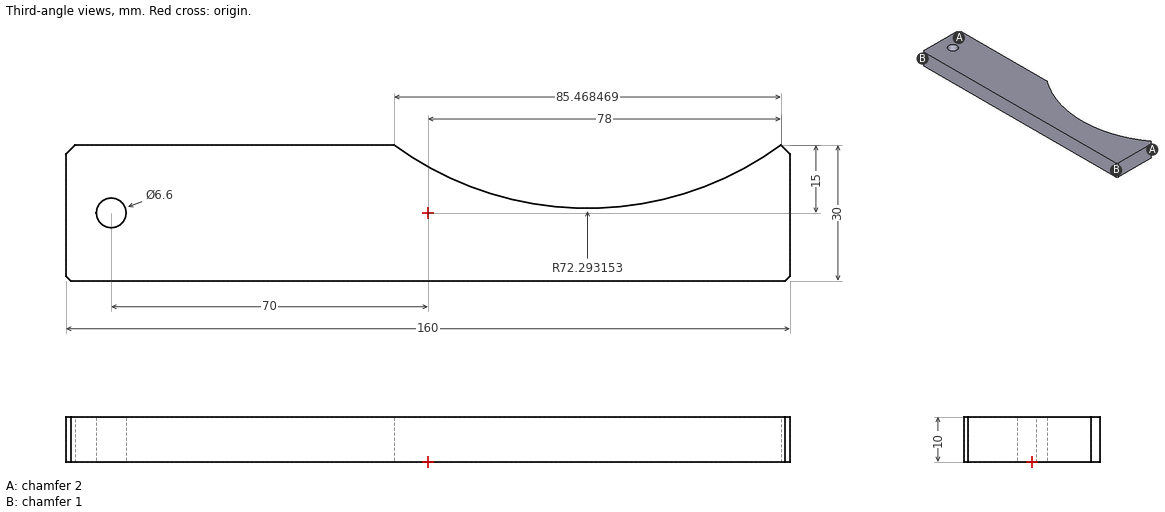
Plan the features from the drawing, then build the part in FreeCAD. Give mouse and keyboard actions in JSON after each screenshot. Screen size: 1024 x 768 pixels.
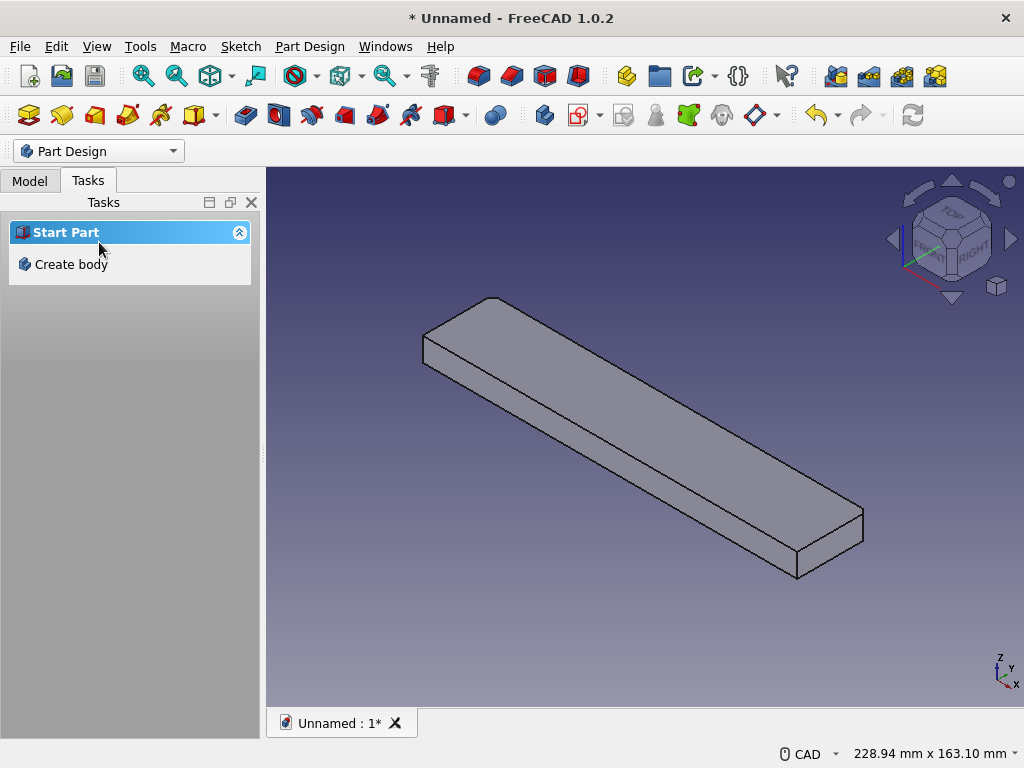
{"action": "left_click", "coordinate": [797, 564]}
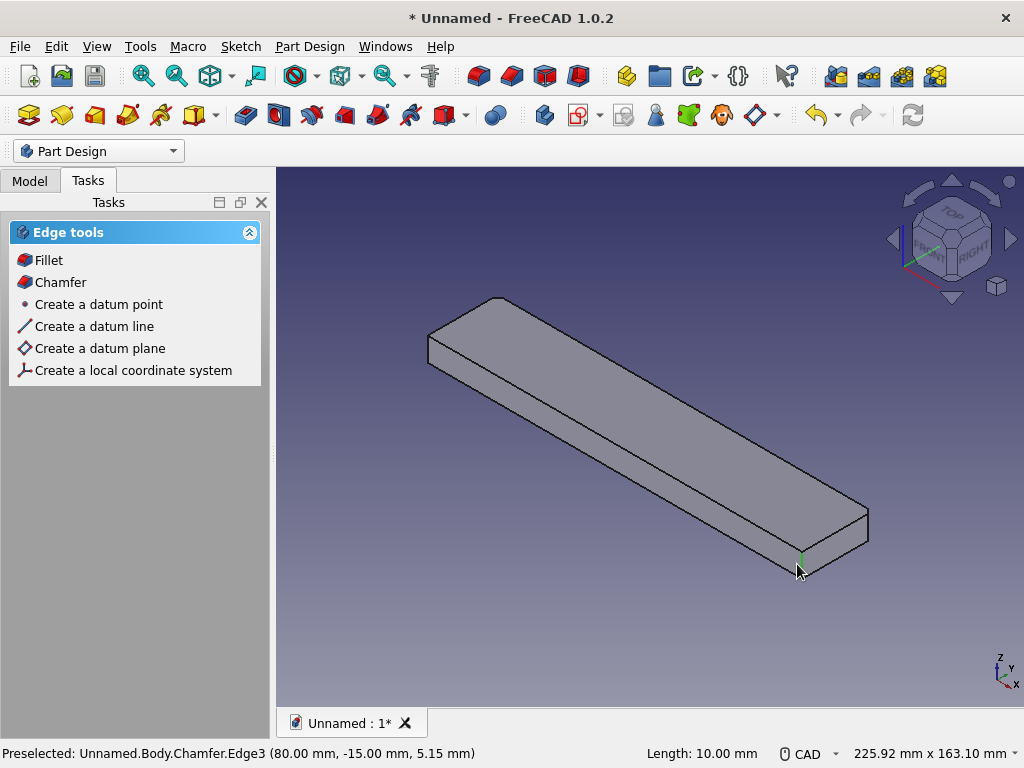
{"action": "key", "text": "2"}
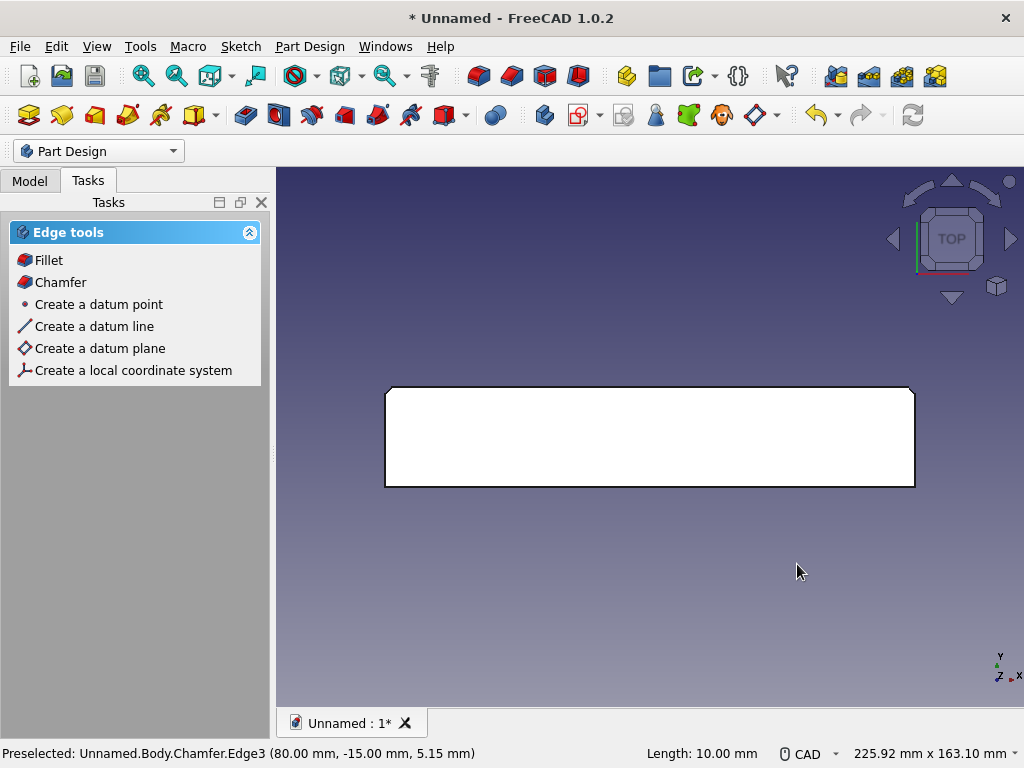
{"action": "key", "text": "1"}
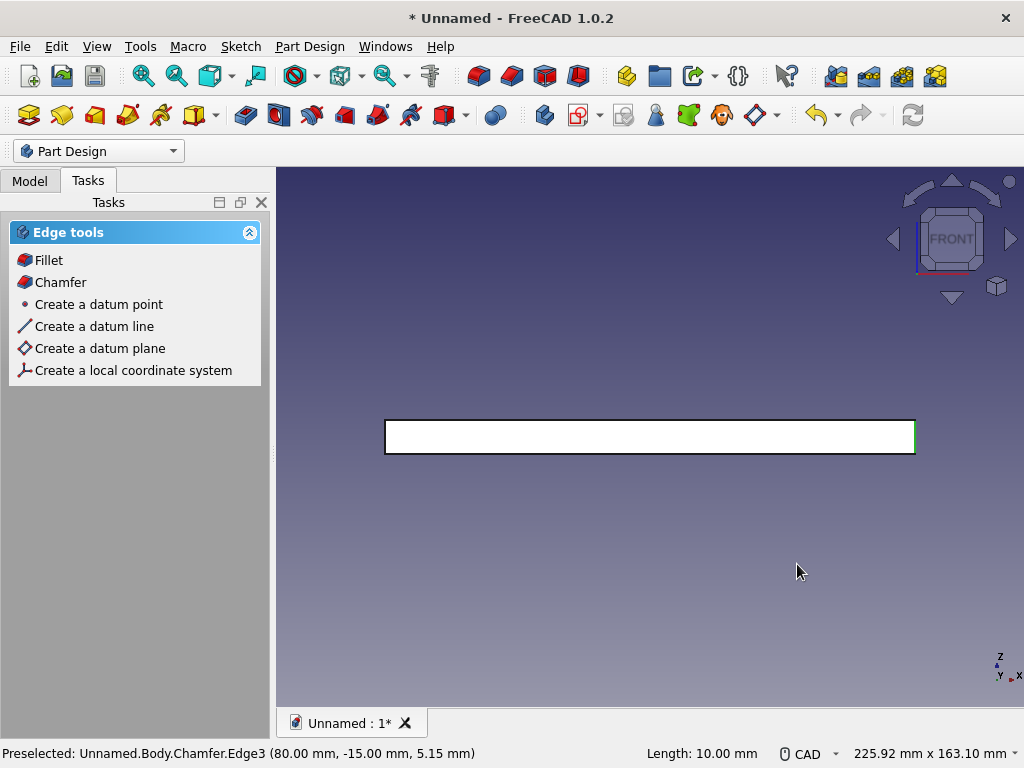
{"action": "left_click", "coordinate": [385, 436], "text": "ctrl"}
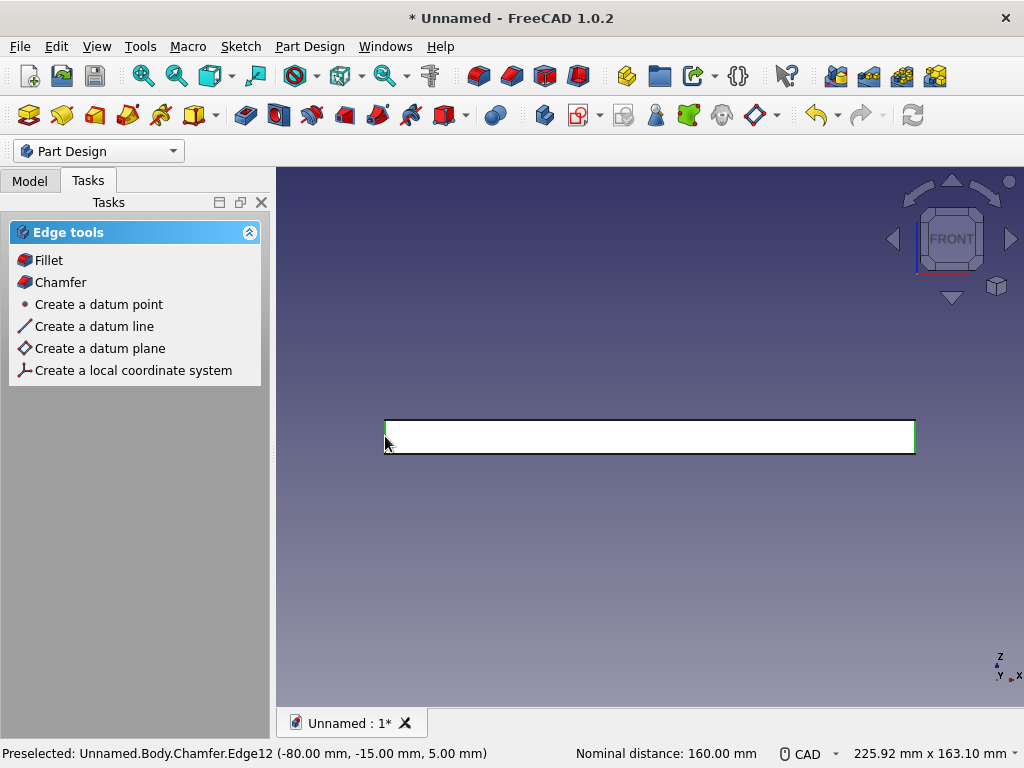
{"action": "left_click", "coordinate": [512, 76]}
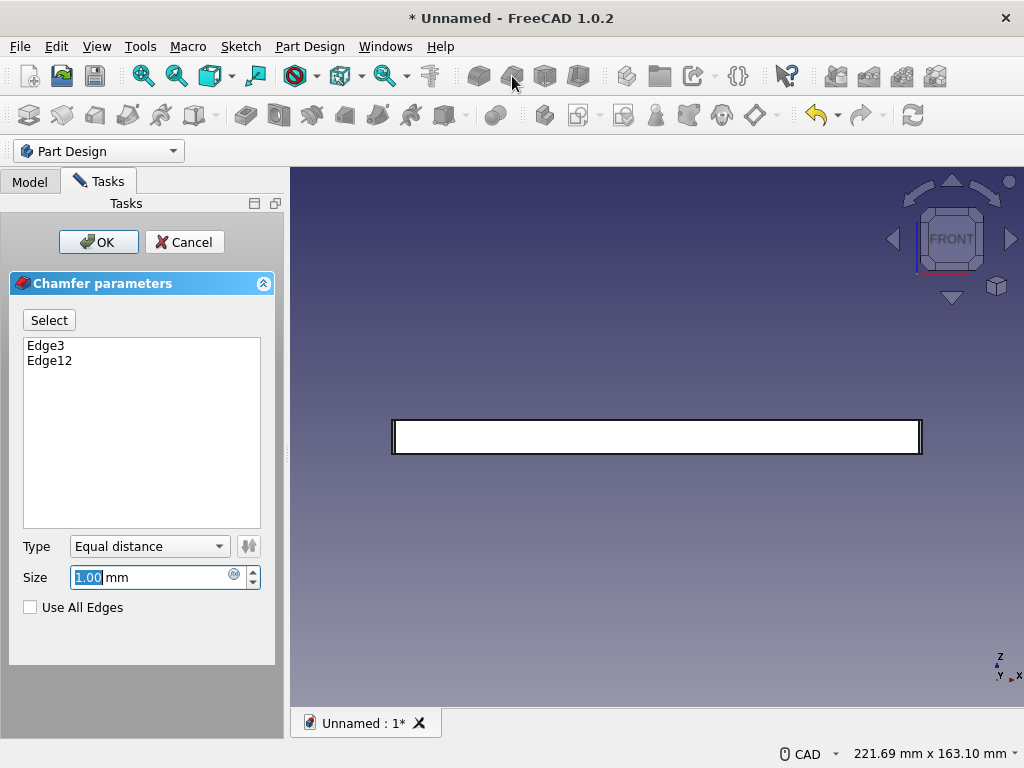
{"action": "type", "text": "1"}
{"action": "key", "text": "Tab"}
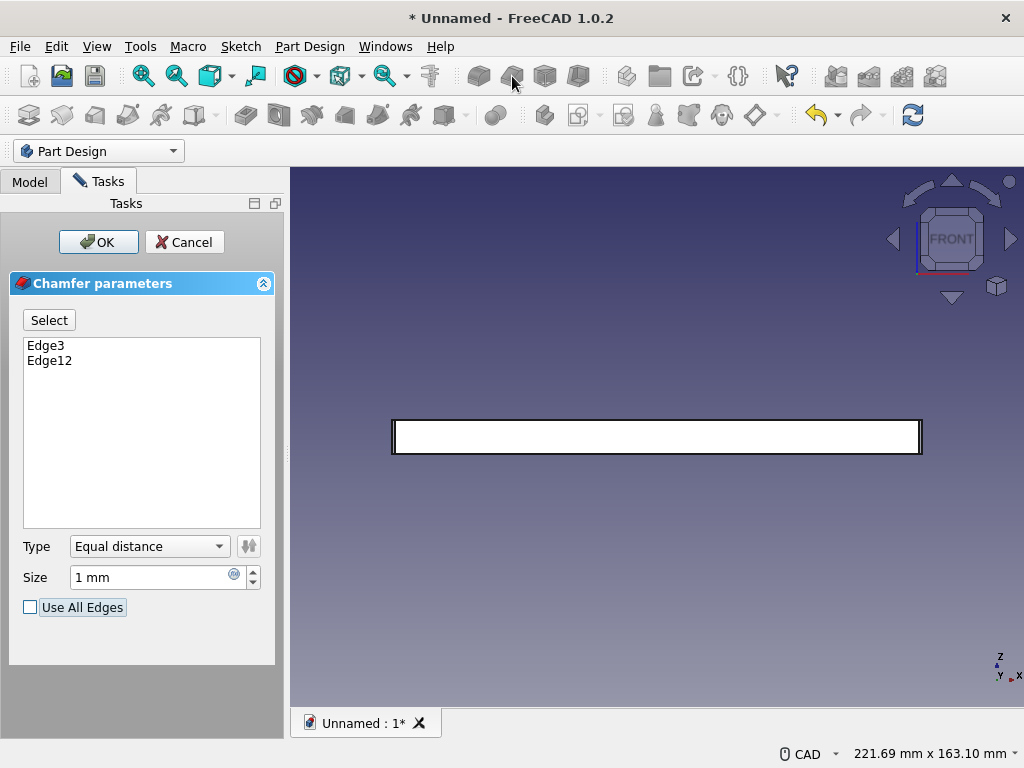
{"action": "left_click", "coordinate": [99, 242]}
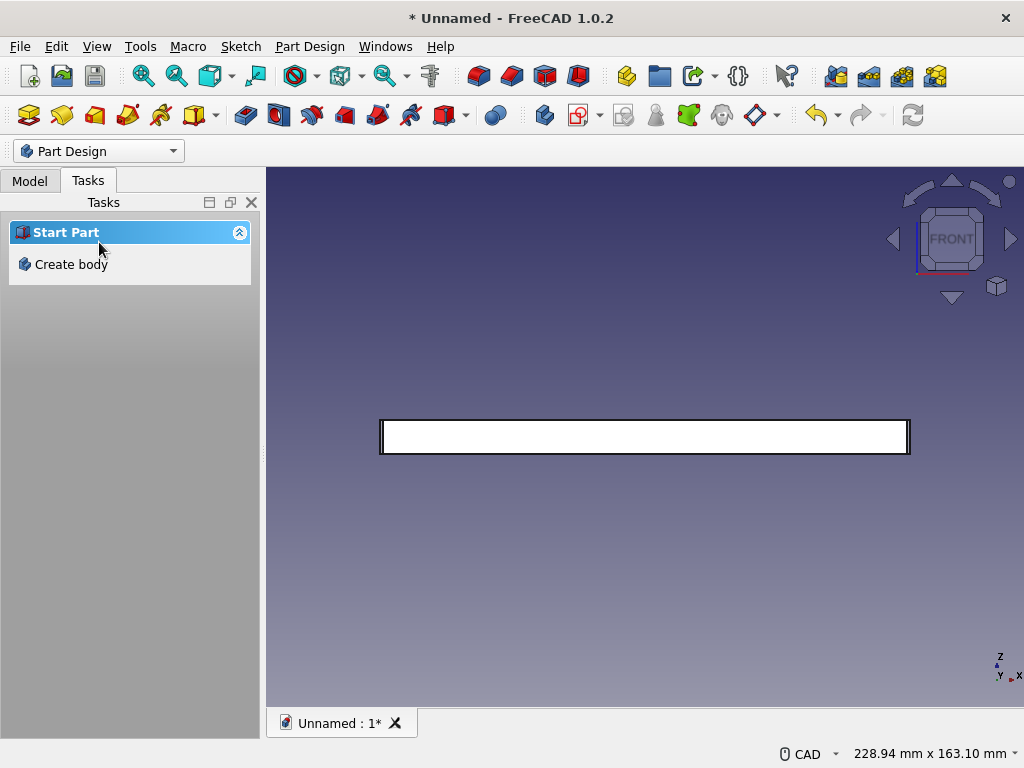
{"action": "key", "text": "0"}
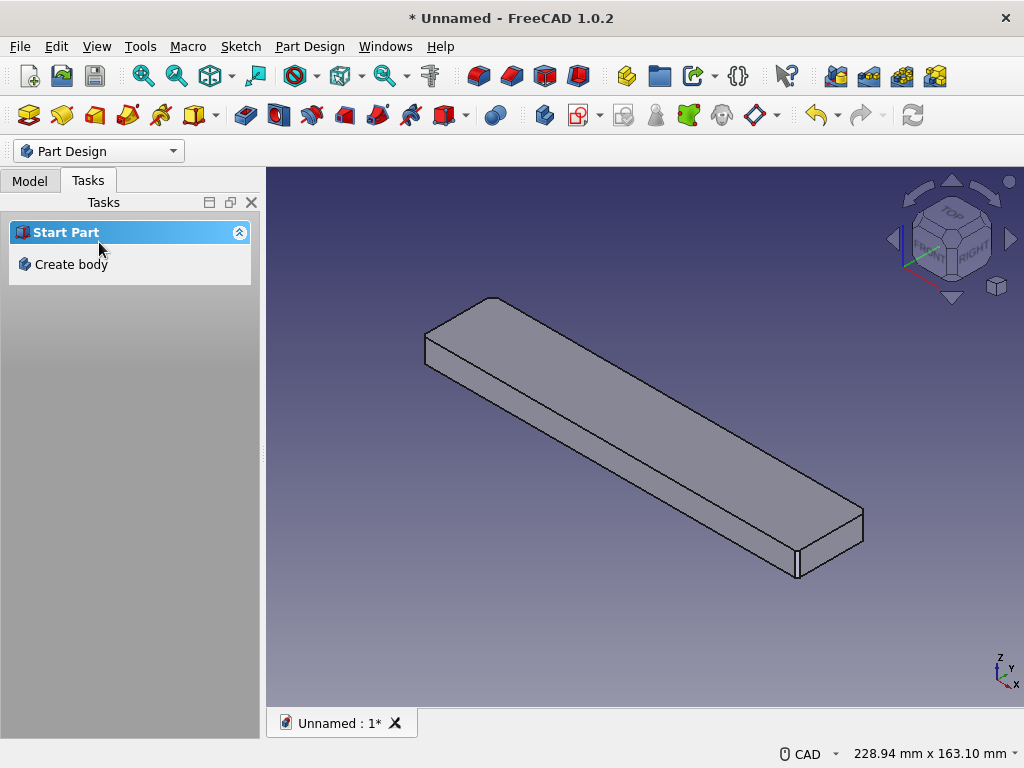
{"action": "left_click", "coordinate": [752, 484]}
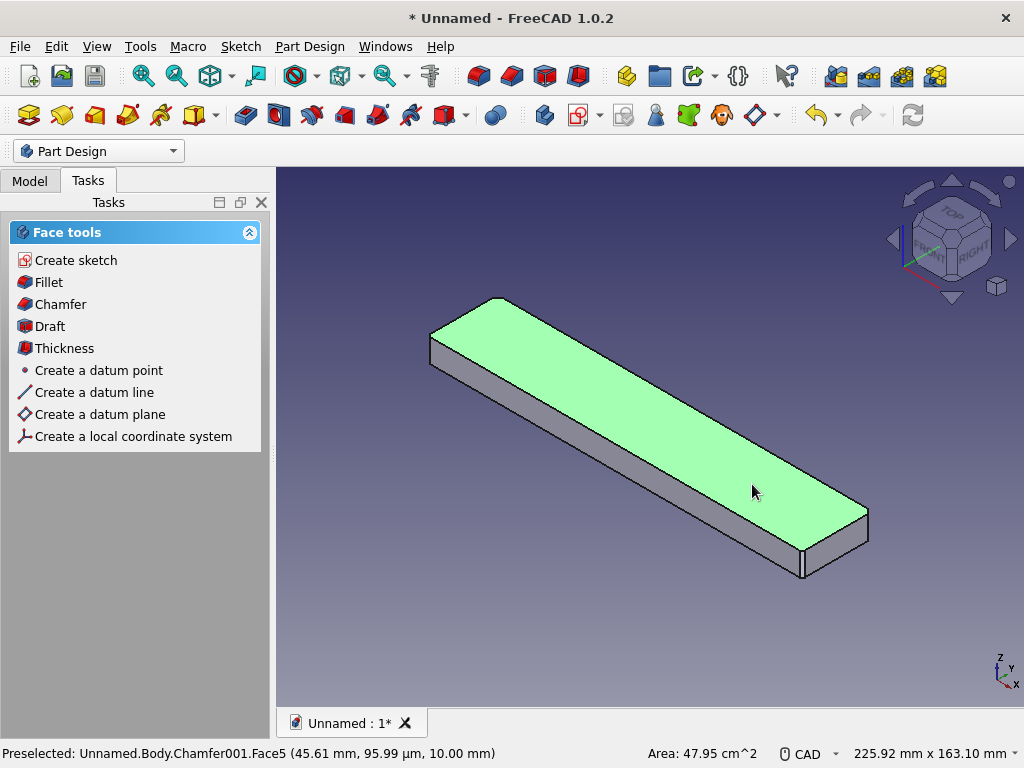
{"action": "left_click", "coordinate": [578, 116]}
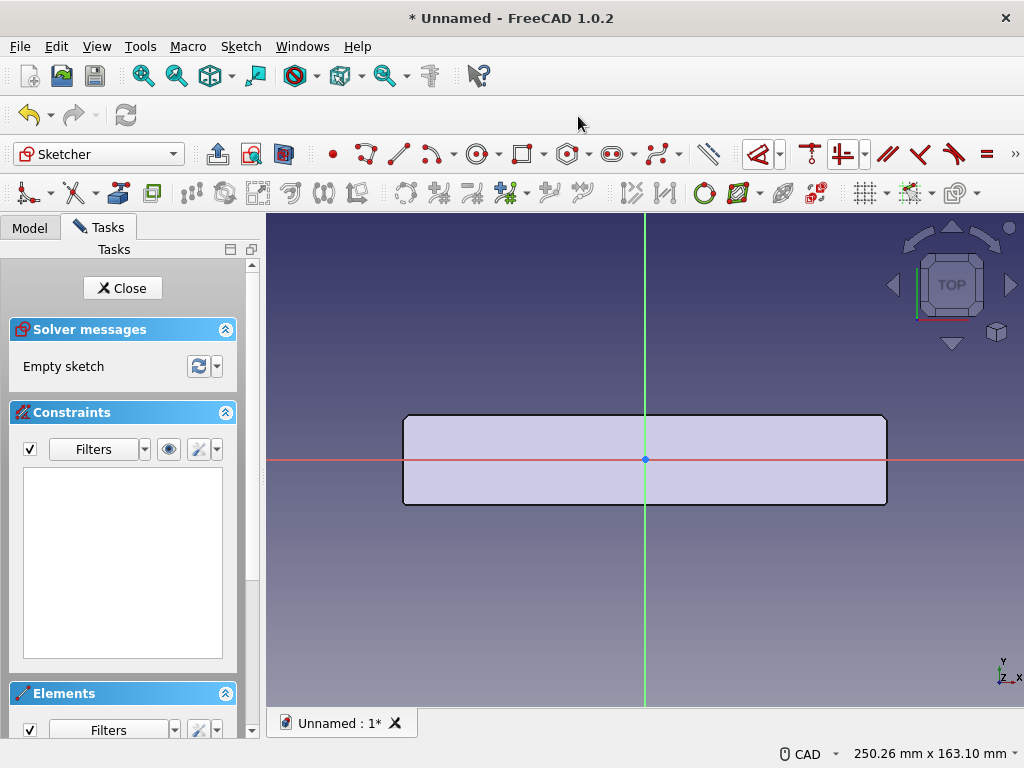
{"action": "scroll", "coordinate": [424, 460], "scroll_direction": "up", "scroll_amount": 14}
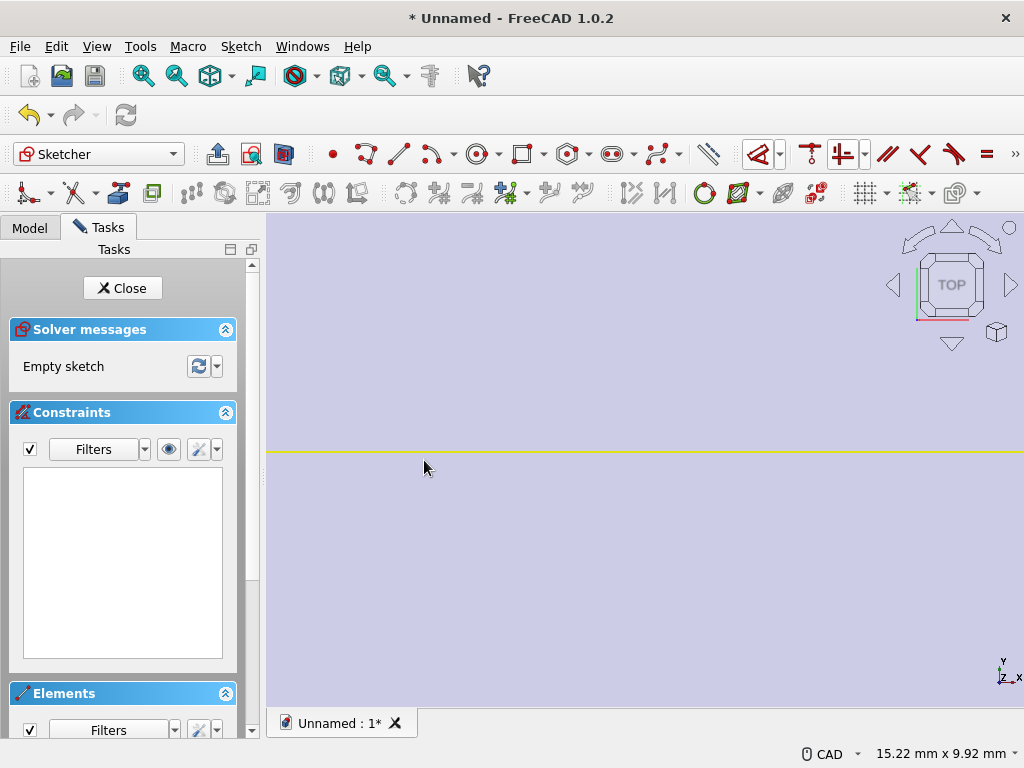
{"action": "left_click", "coordinate": [476, 154]}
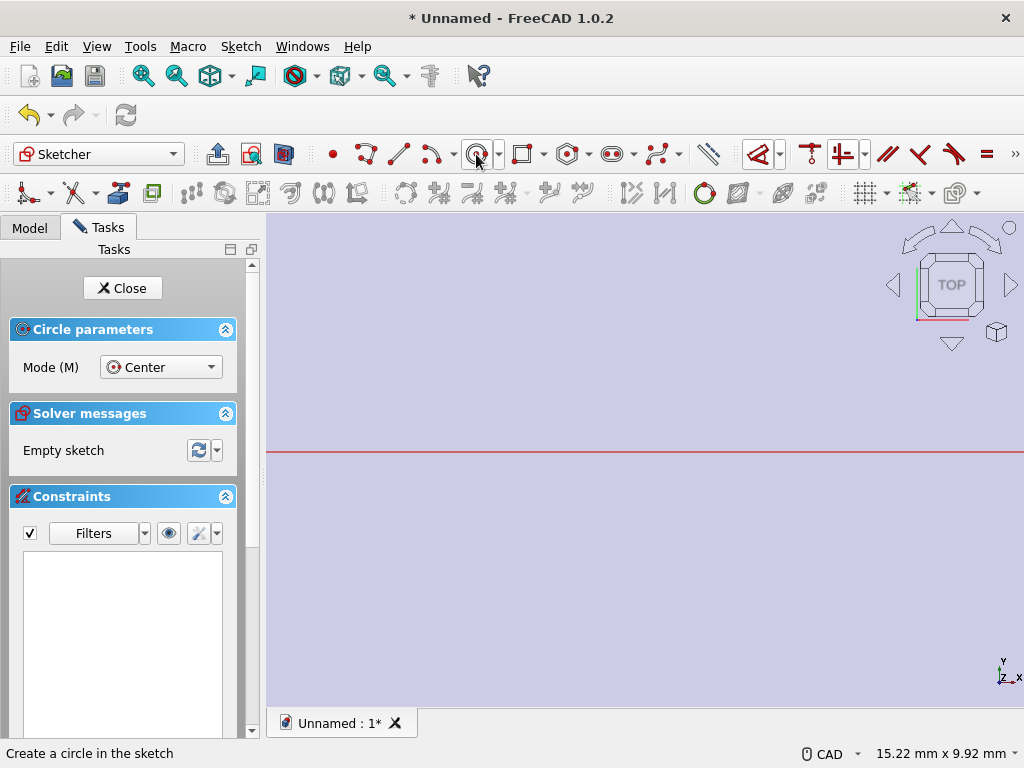
{"action": "left_click", "coordinate": [568, 452]}
{"action": "mouse_move", "coordinate": [685, 336]}